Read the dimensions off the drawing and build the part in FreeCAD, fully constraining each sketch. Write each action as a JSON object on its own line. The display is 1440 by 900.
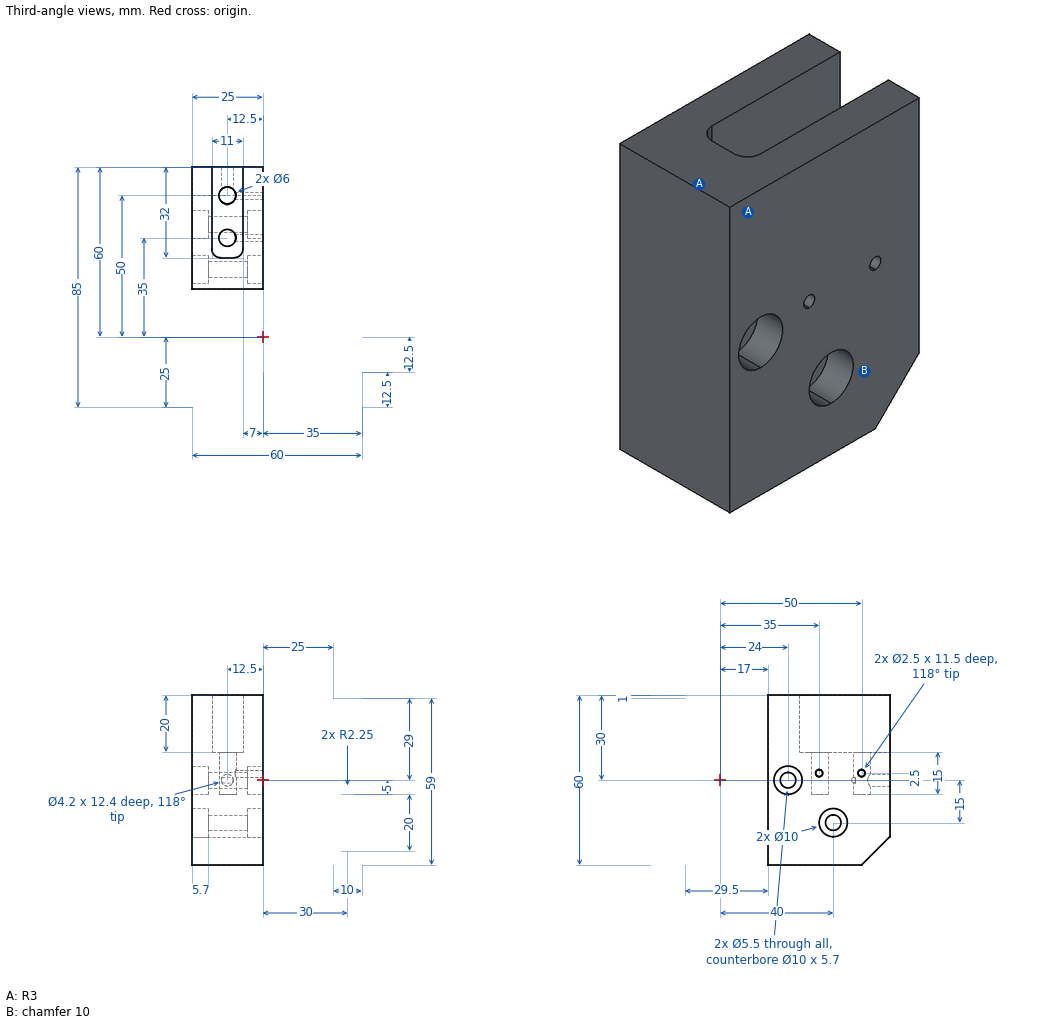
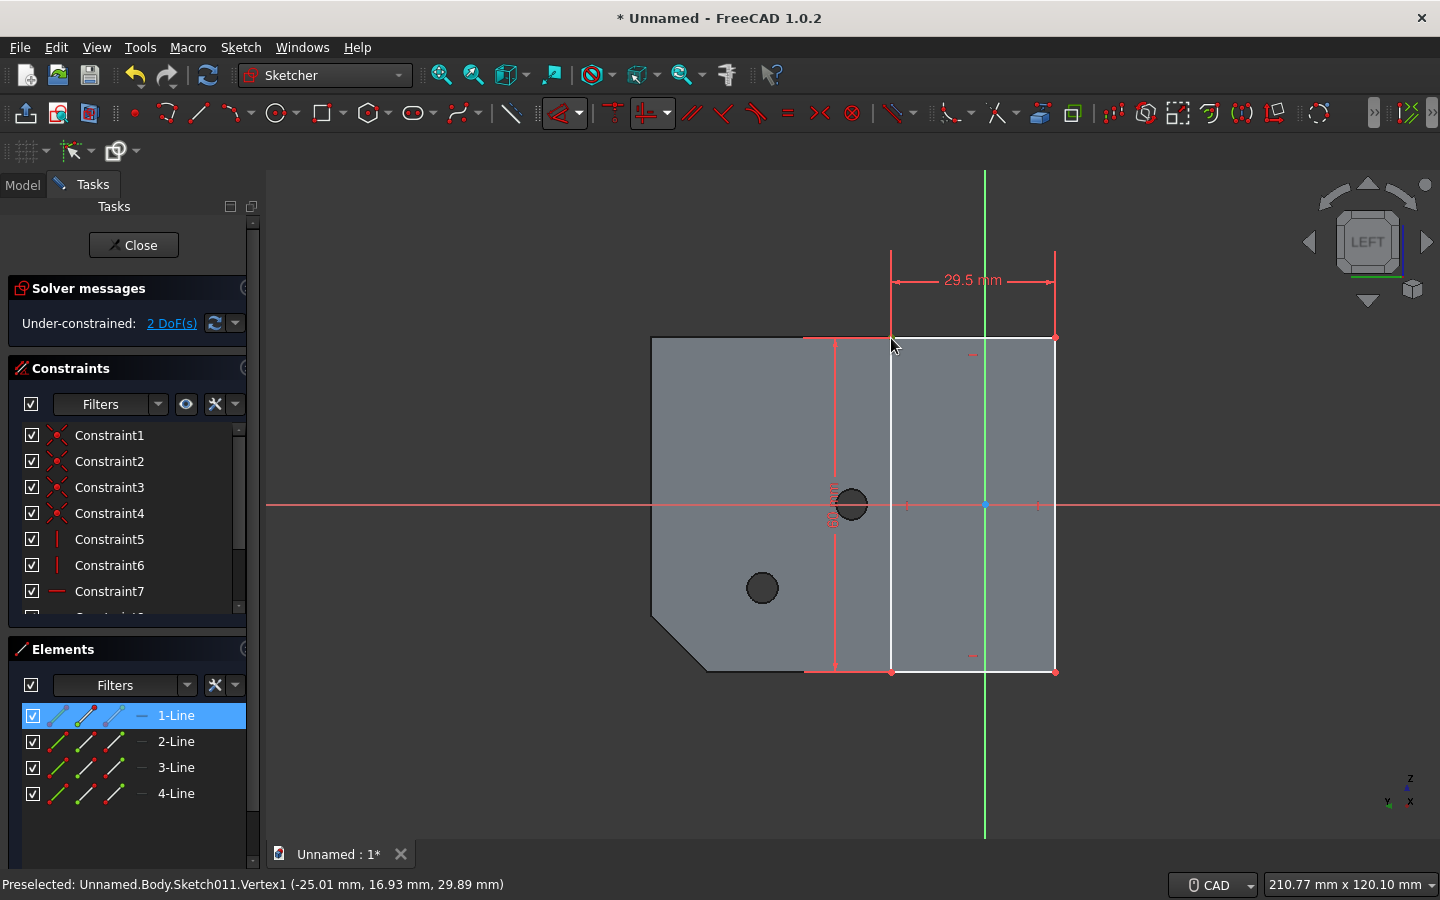
{"action": "key", "text": "l"}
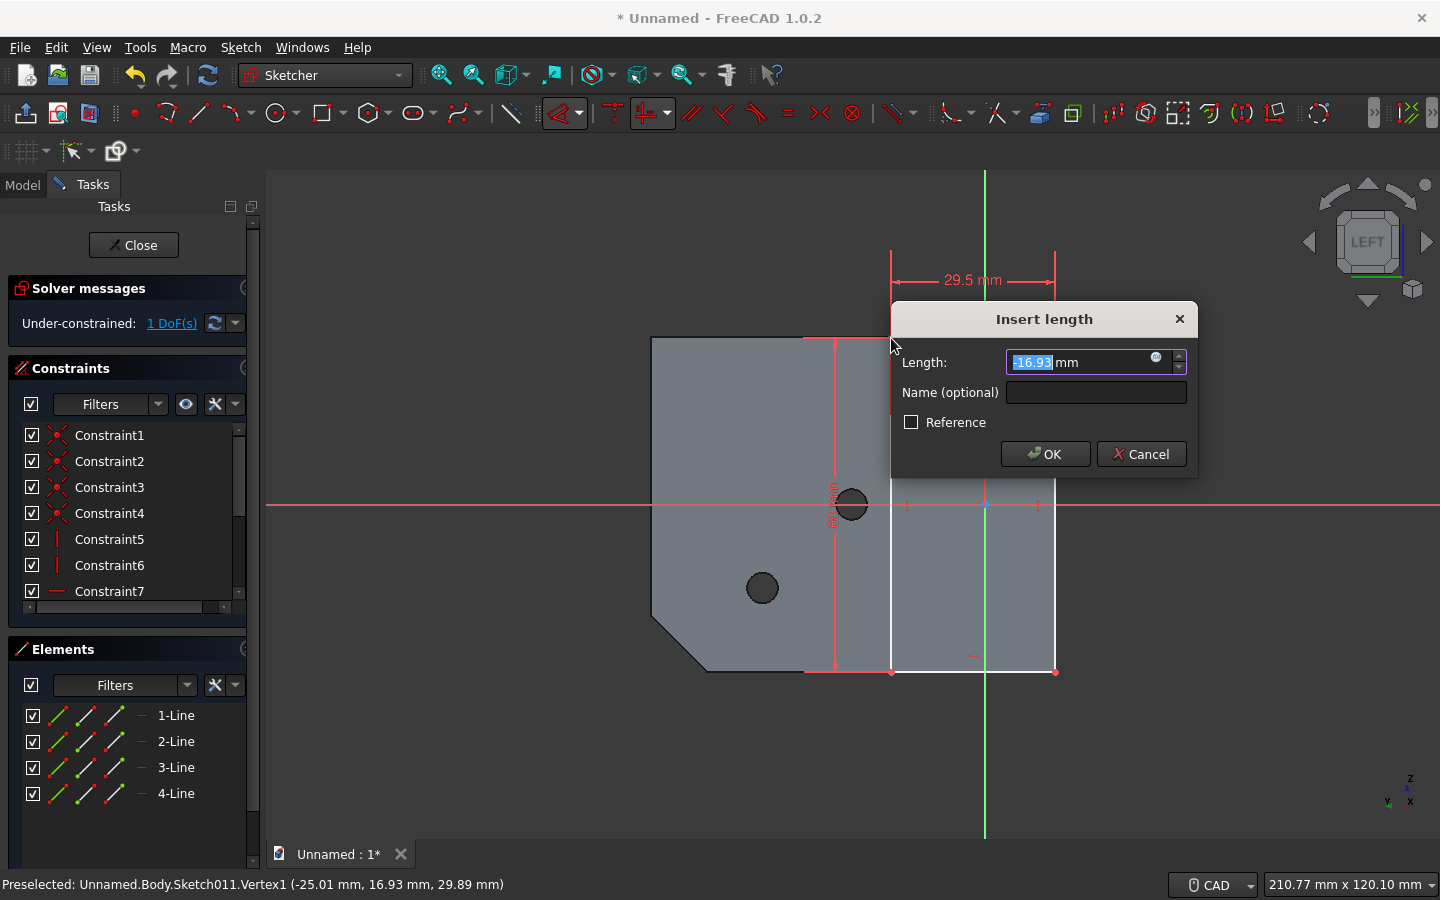
{"action": "type", "text": "-17"}
{"action": "key", "text": "Return"}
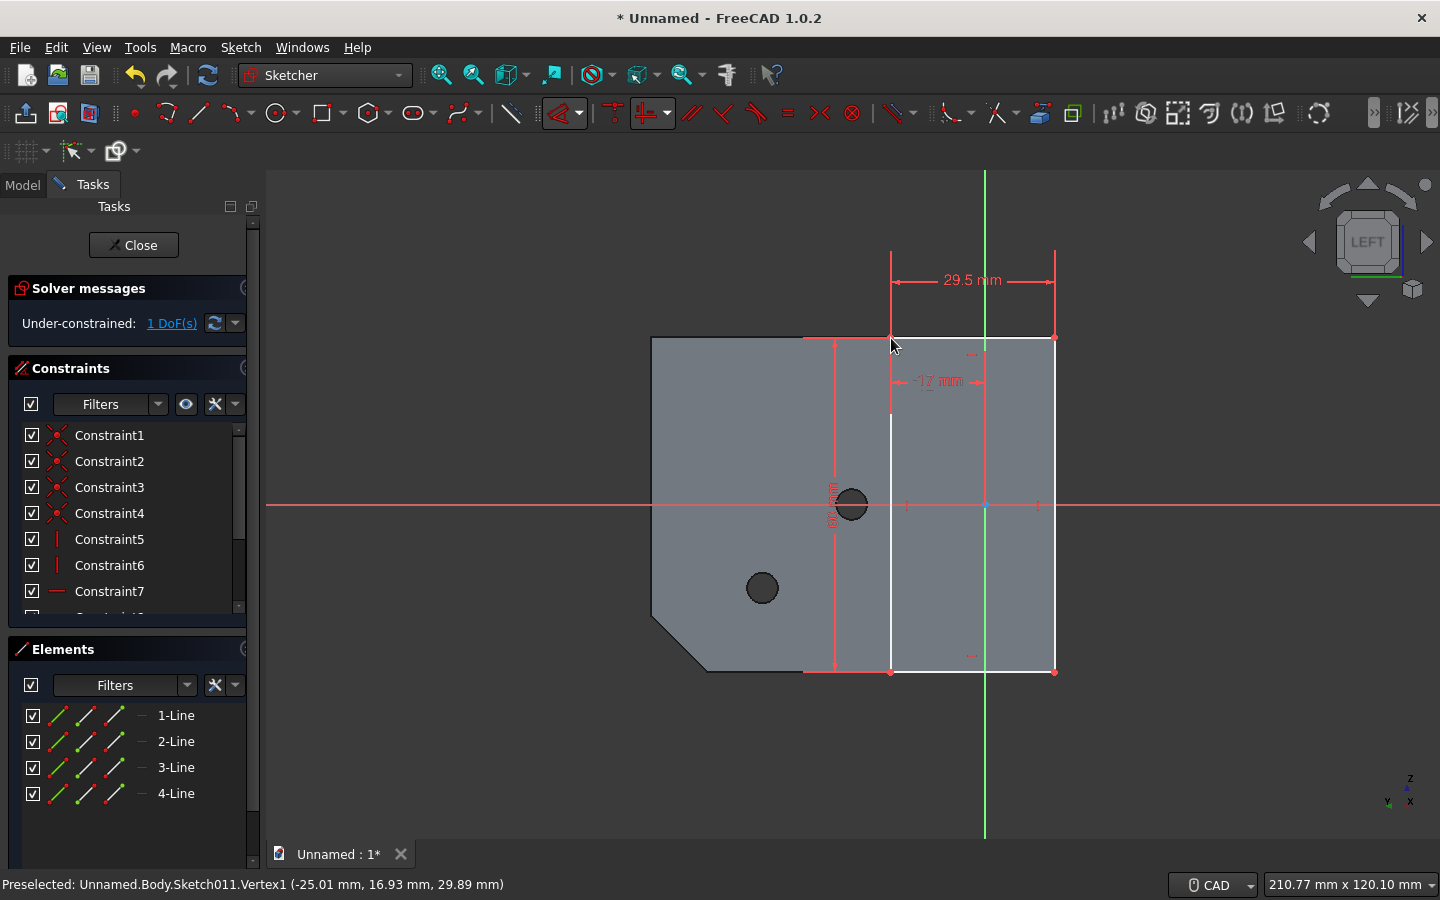
{"action": "left_click", "coordinate": [891, 338]}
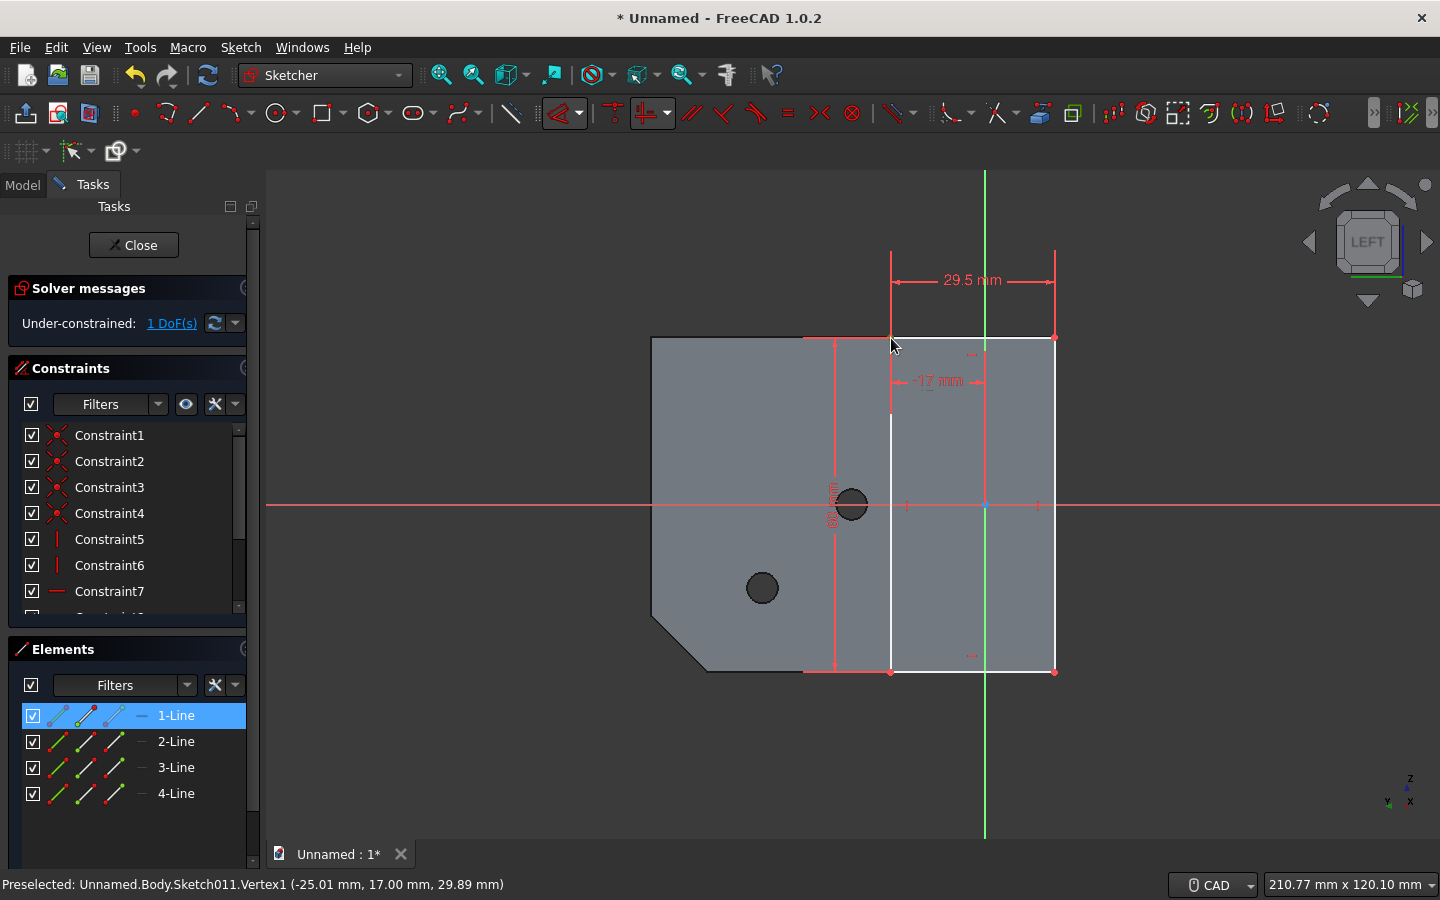
{"action": "key", "text": "i"}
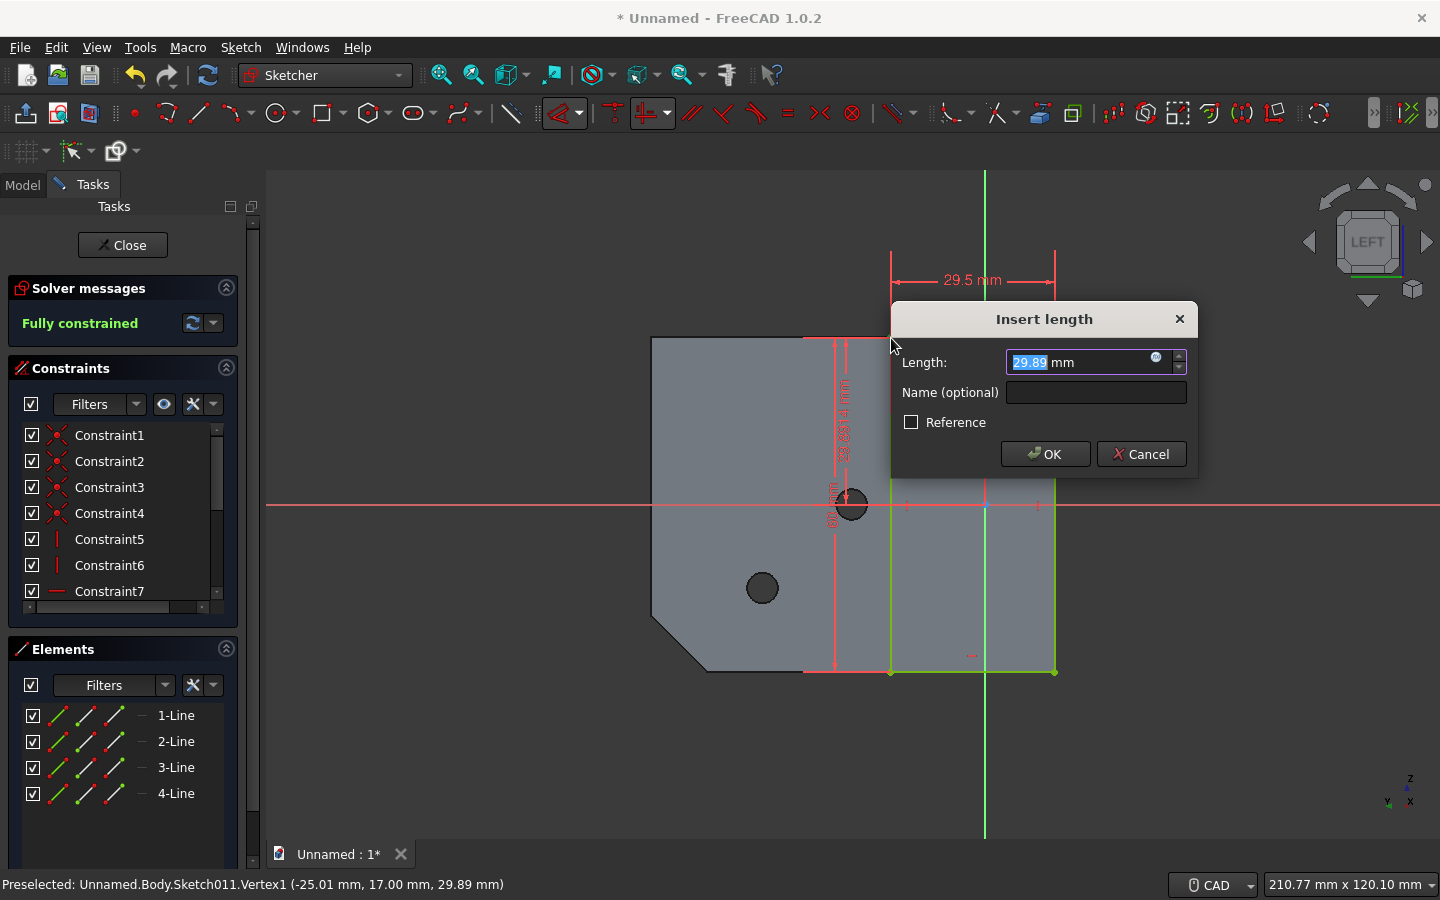
{"action": "type", "text": "30"}
{"action": "key", "text": "Return"}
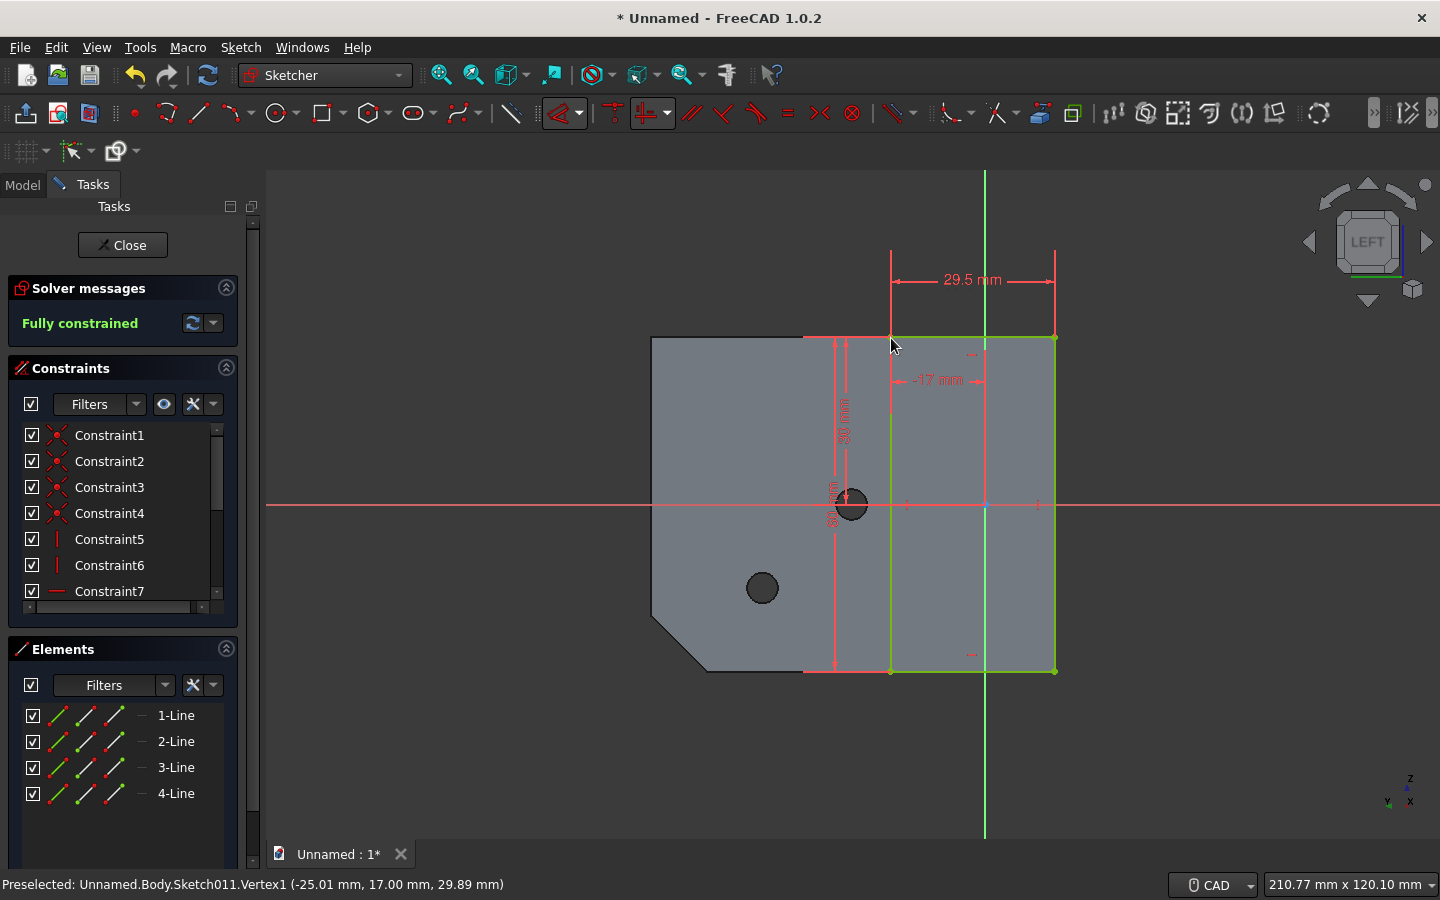
{"action": "left_click", "coordinate": [123, 245]}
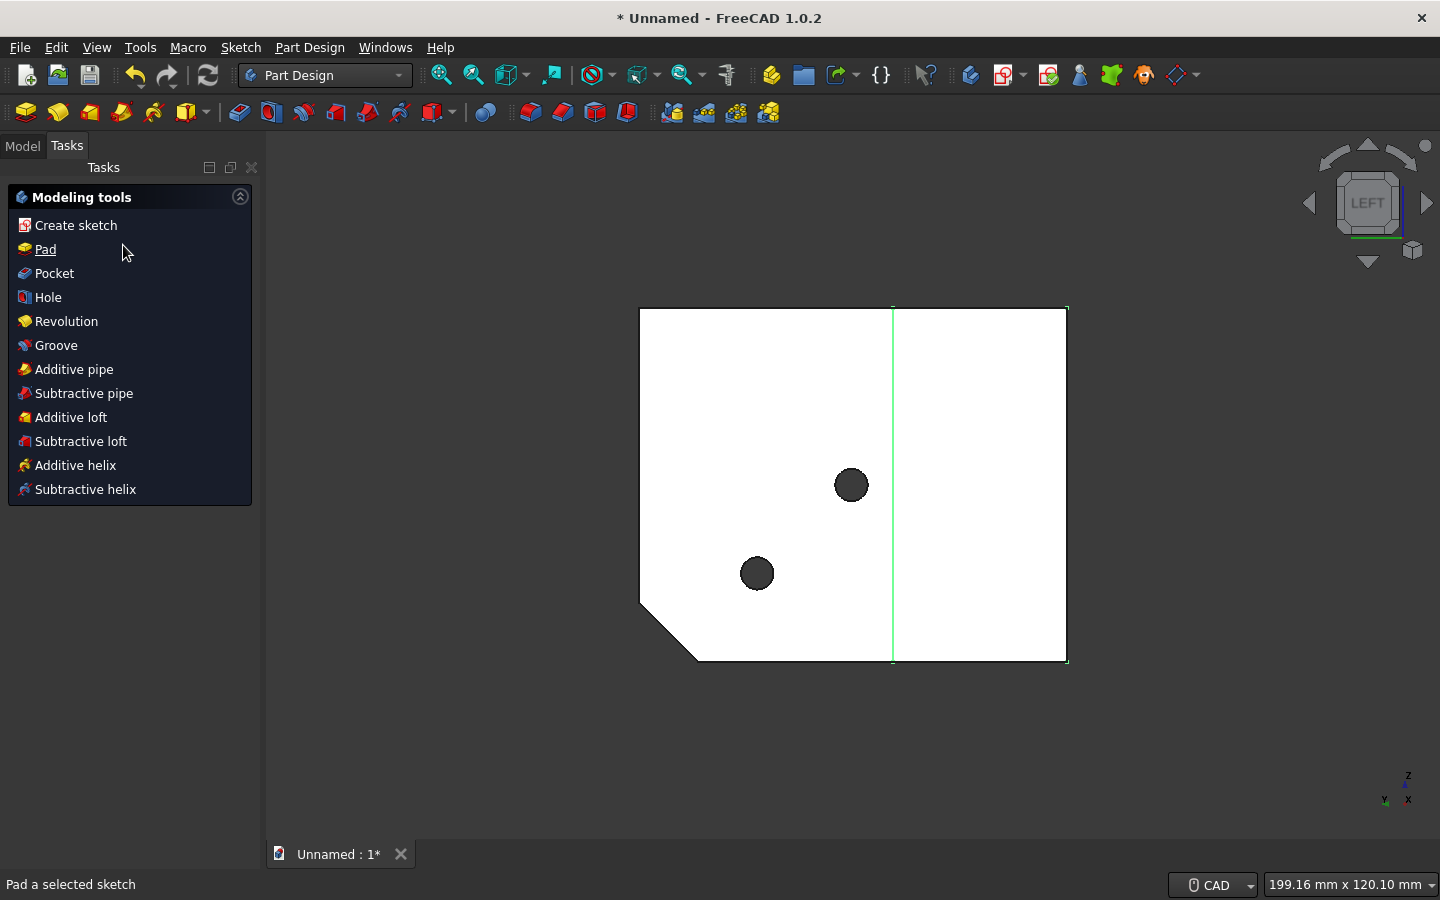
{"action": "left_click", "coordinate": [240, 112]}